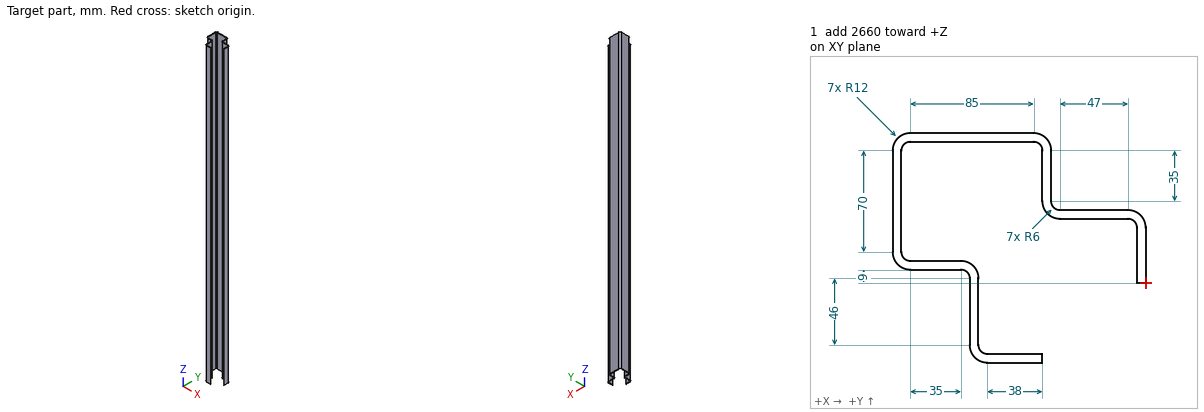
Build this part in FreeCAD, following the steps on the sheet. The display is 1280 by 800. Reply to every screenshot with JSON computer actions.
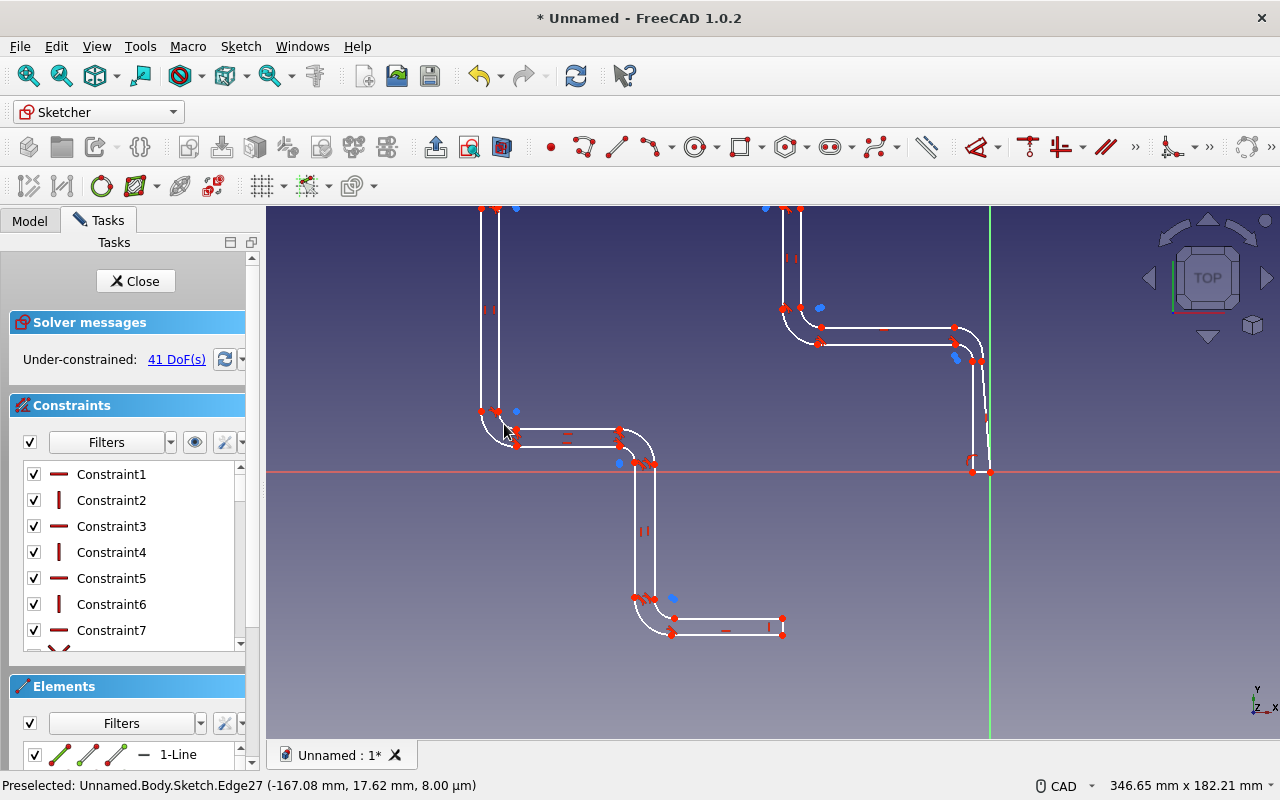
{"action": "left_click", "coordinate": [499, 350]}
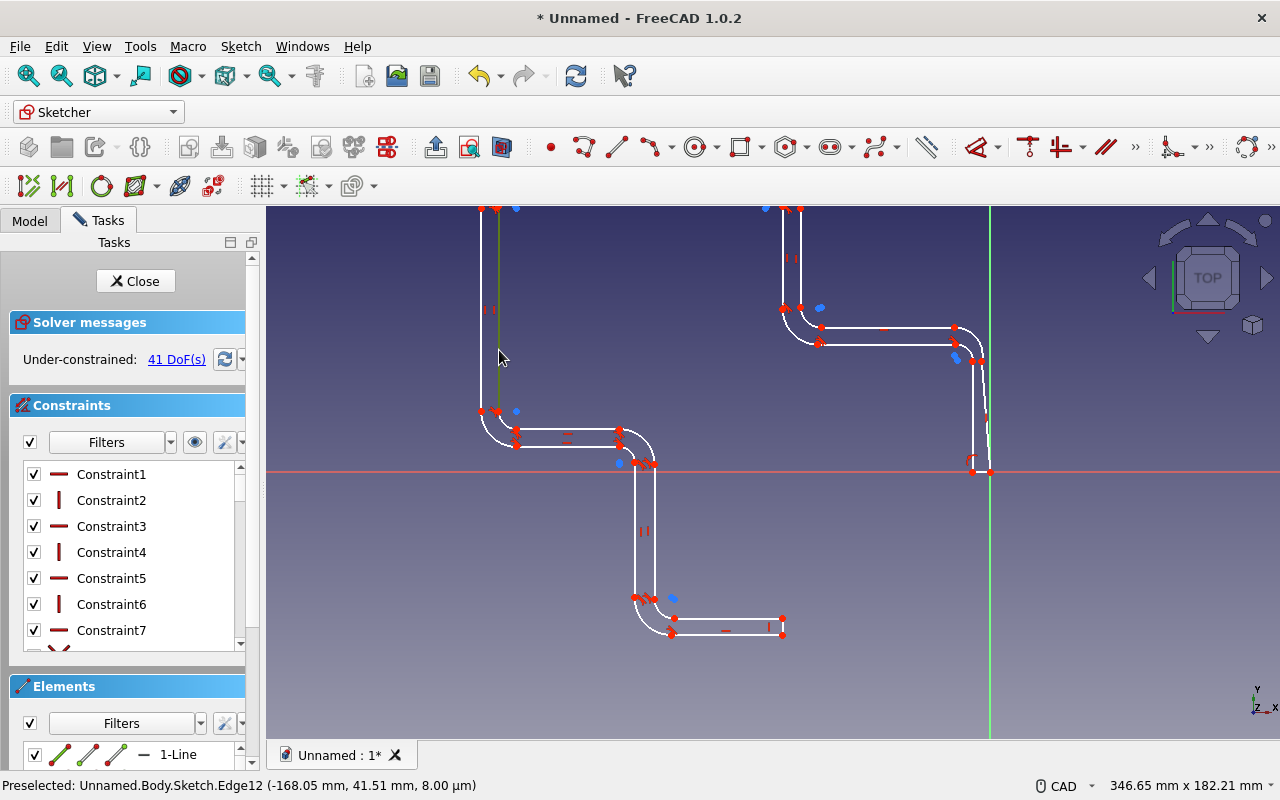
{"action": "left_click", "coordinate": [504, 424]}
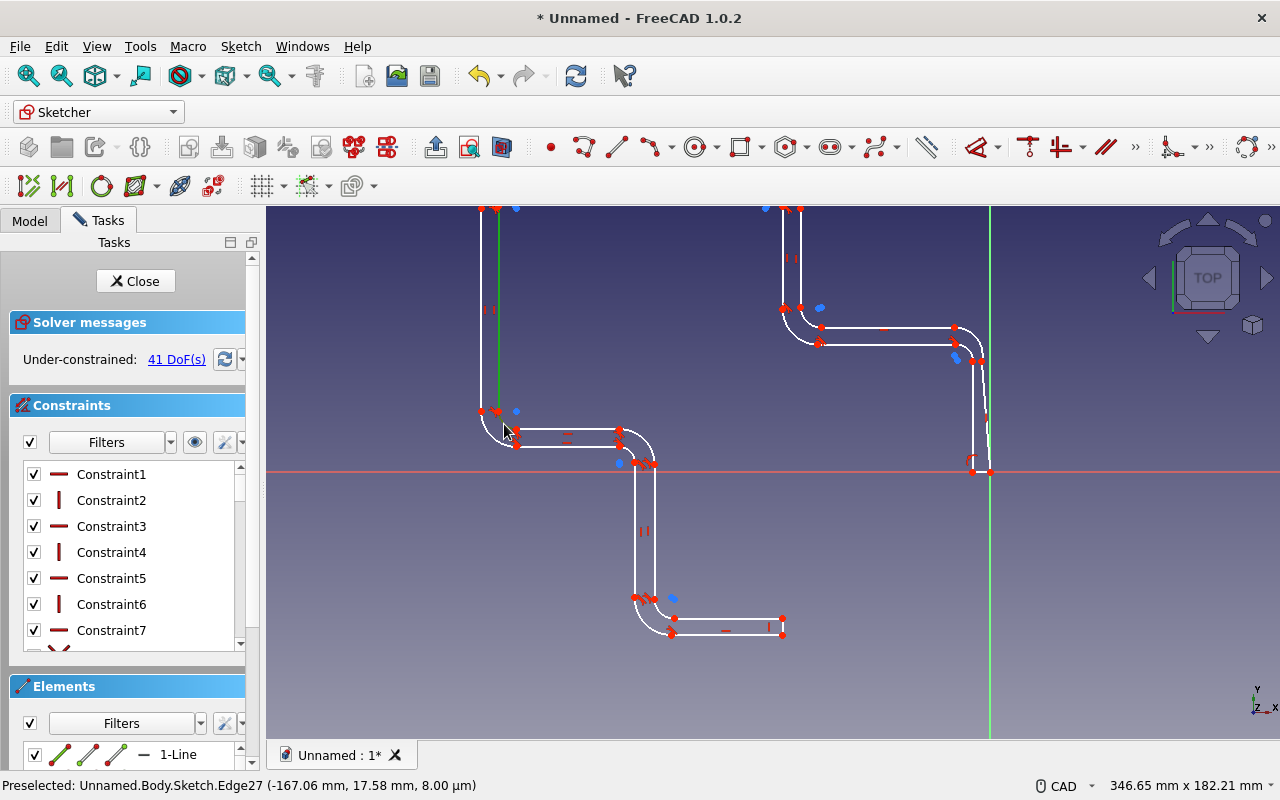
{"action": "key", "text": "t"}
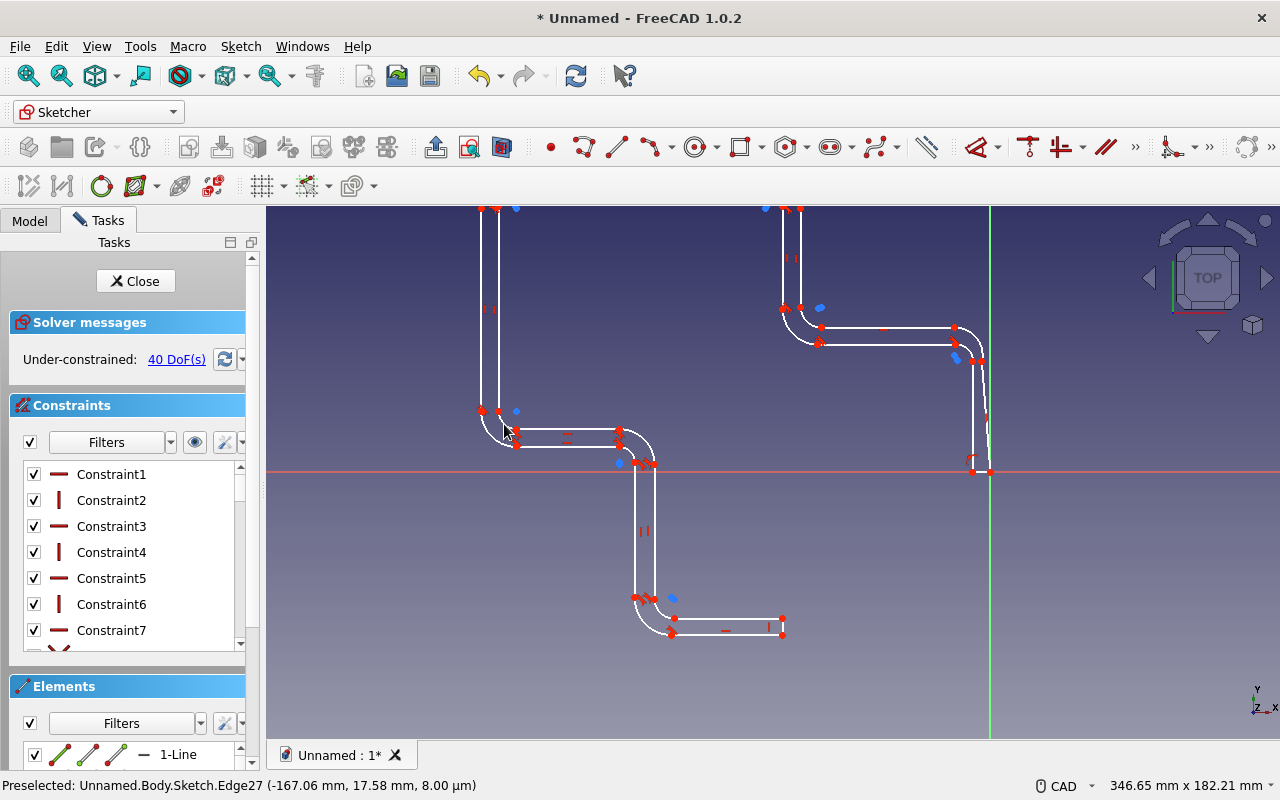
{"action": "left_click", "coordinate": [499, 350]}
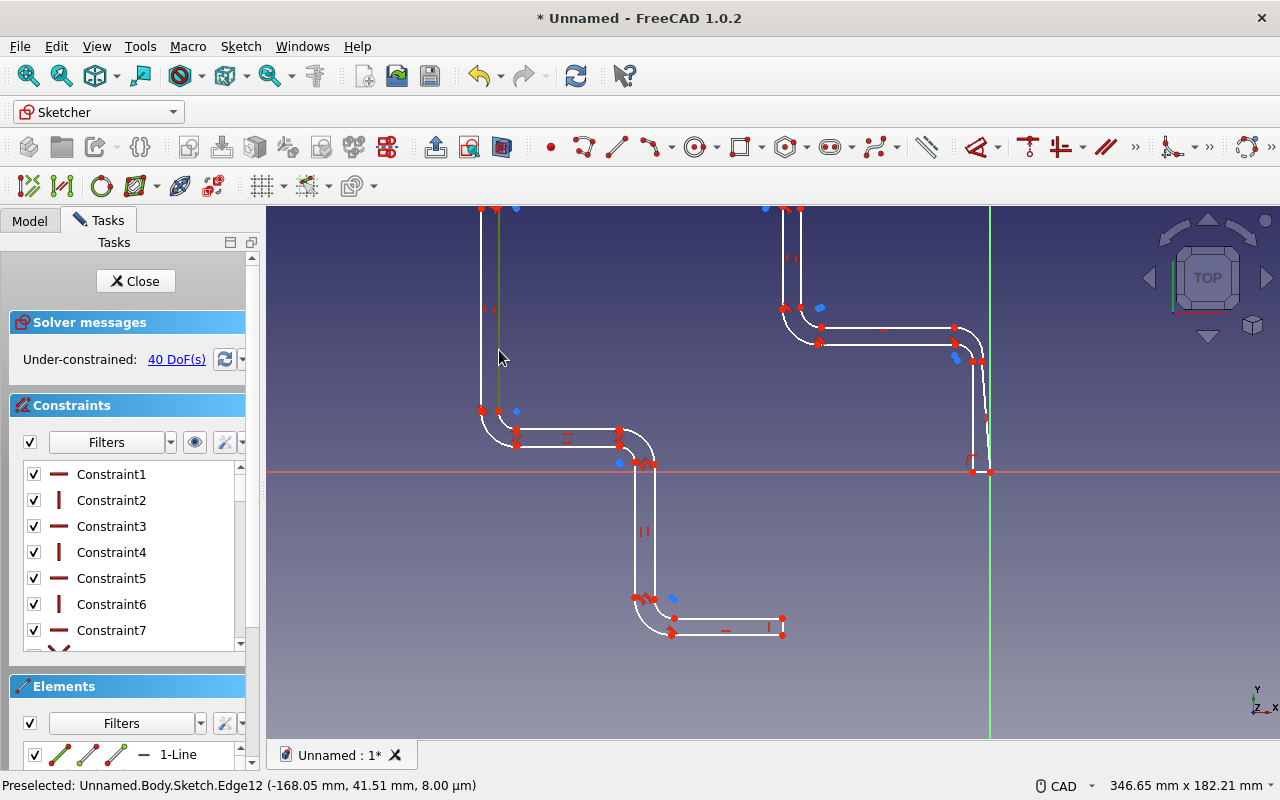
{"action": "scroll", "coordinate": [640, 615], "scroll_direction": "down", "scroll_amount": 2}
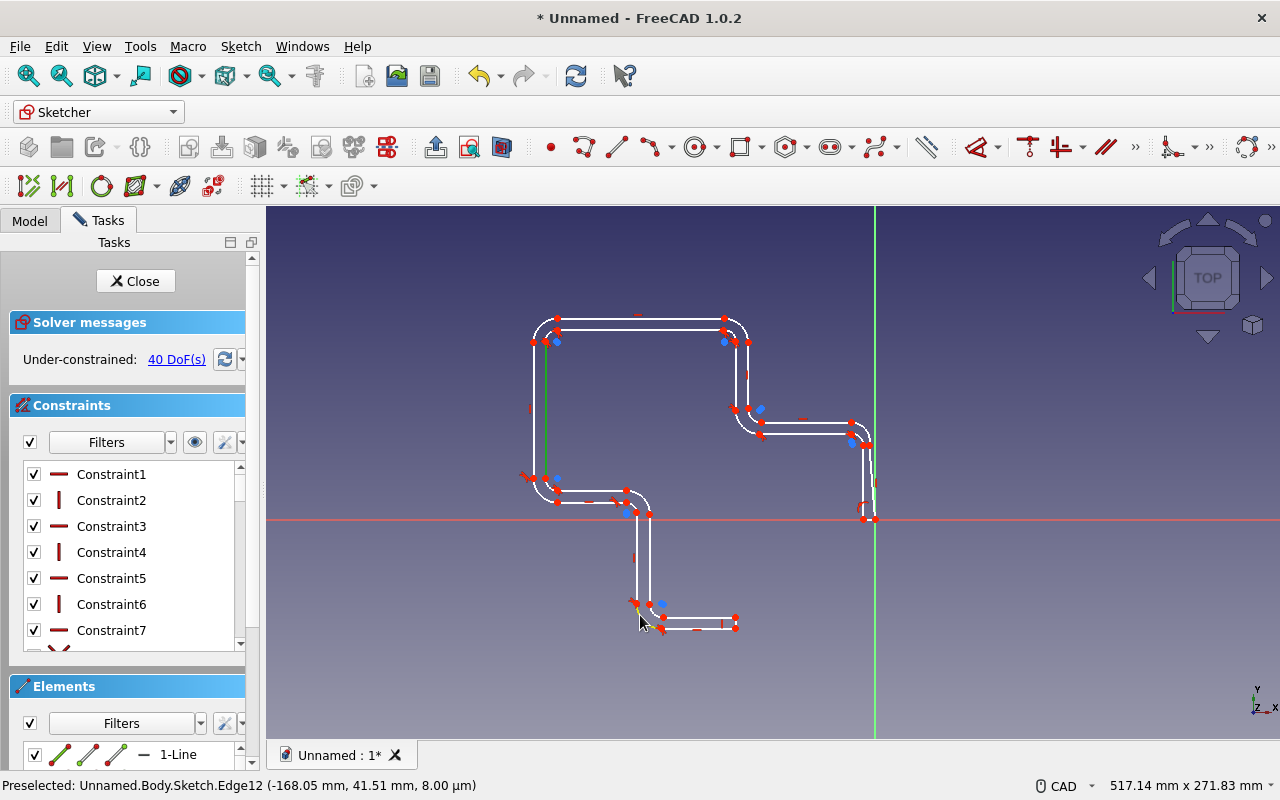
{"action": "scroll", "coordinate": [549, 333], "scroll_direction": "up", "scroll_amount": 3}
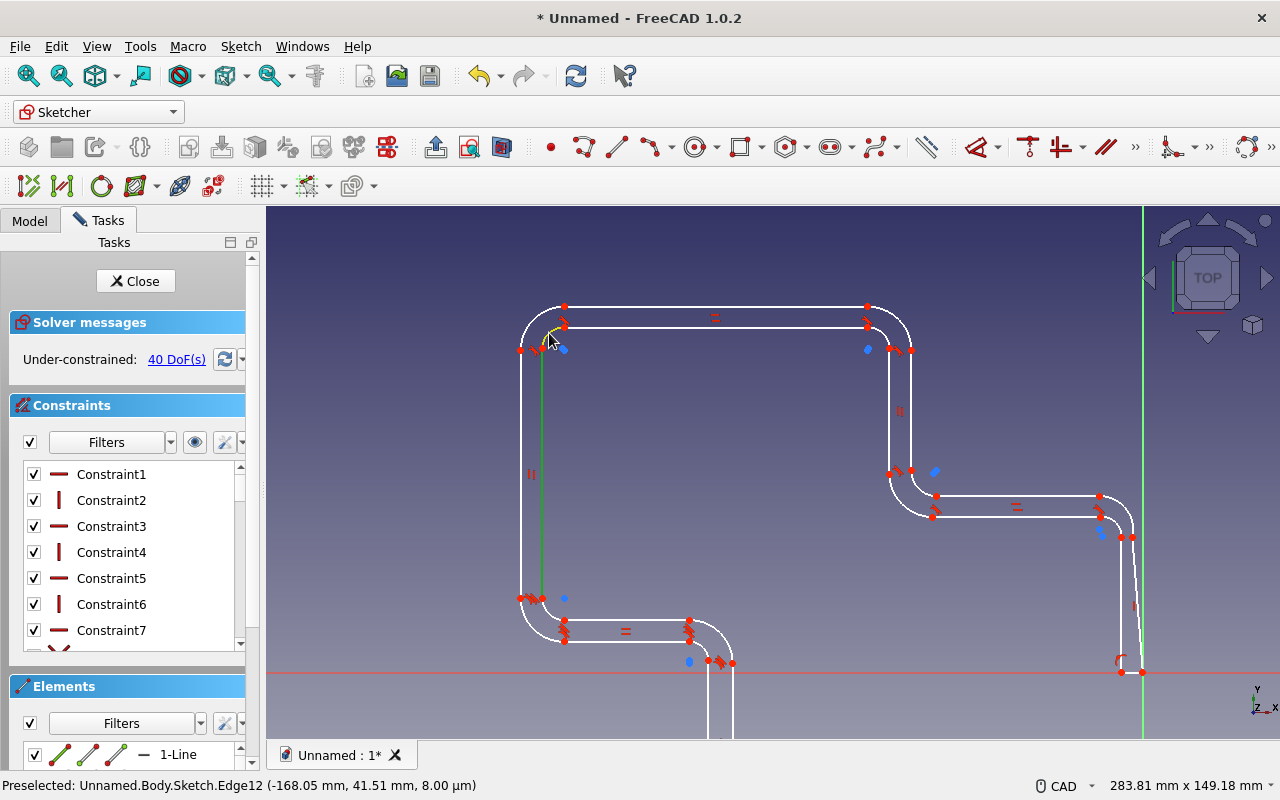
{"action": "left_click", "coordinate": [549, 333]}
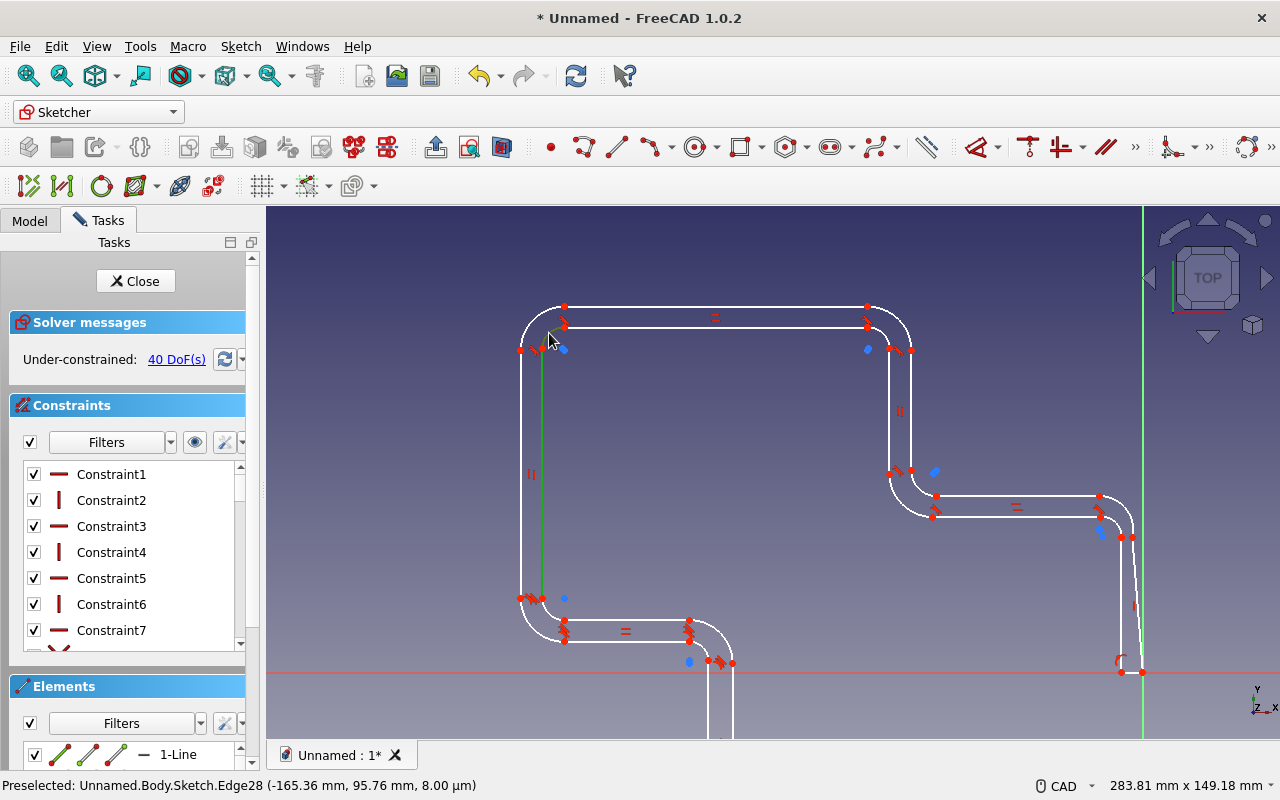
{"action": "key", "text": "t"}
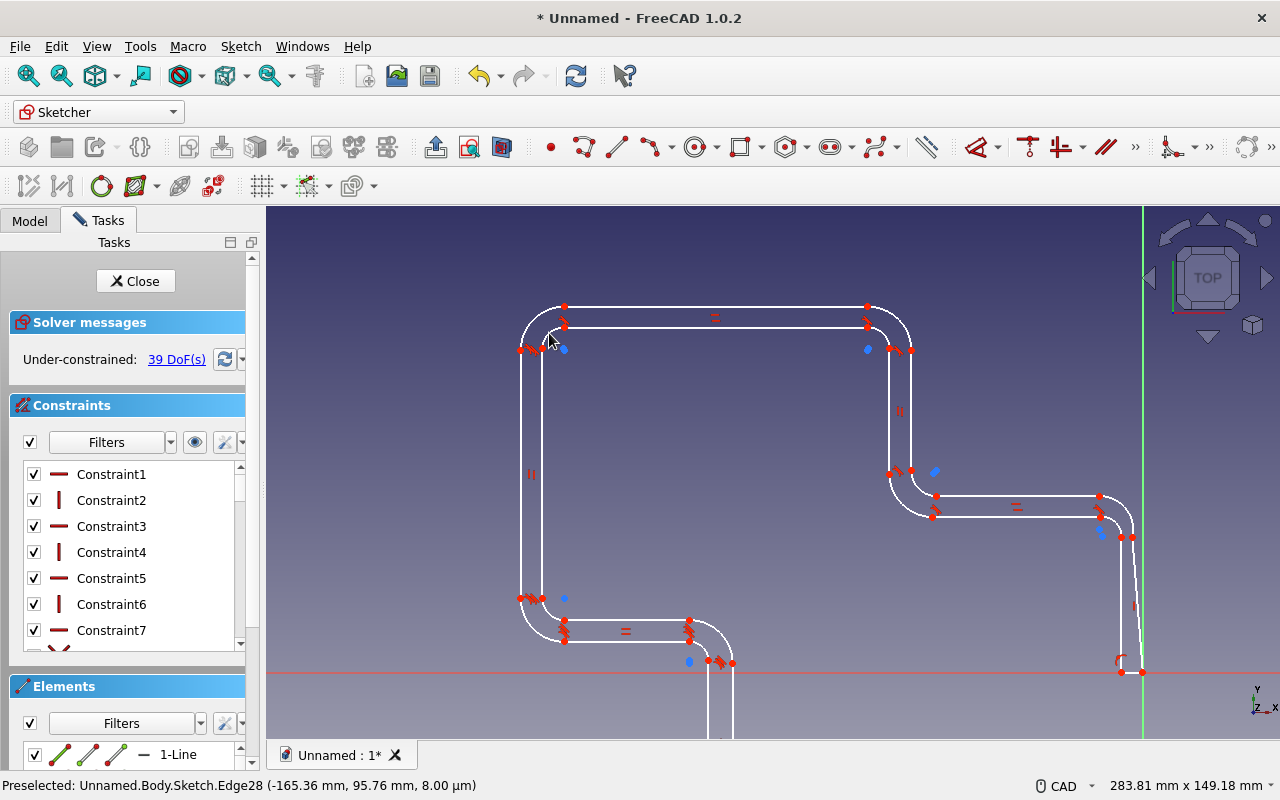
{"action": "left_click", "coordinate": [655, 328]}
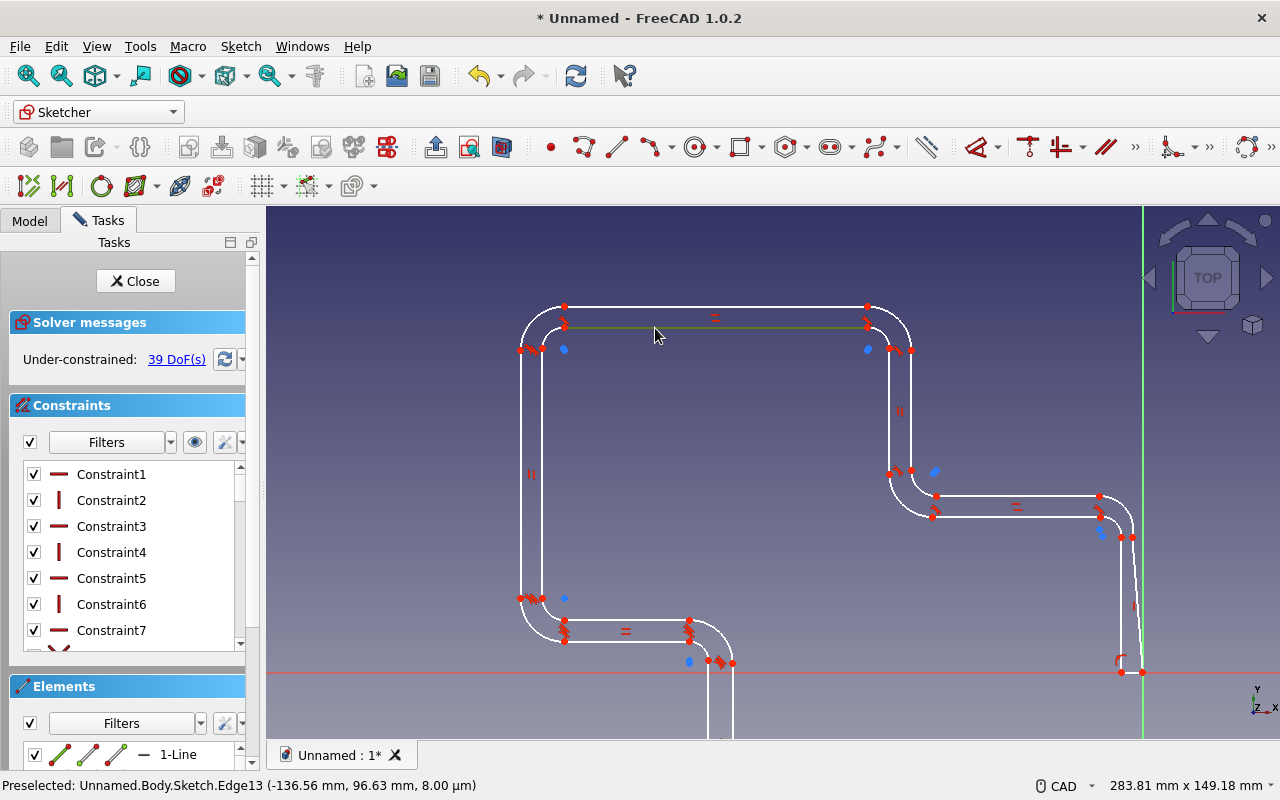
{"action": "scroll", "coordinate": [555, 330], "scroll_direction": "up", "scroll_amount": 2}